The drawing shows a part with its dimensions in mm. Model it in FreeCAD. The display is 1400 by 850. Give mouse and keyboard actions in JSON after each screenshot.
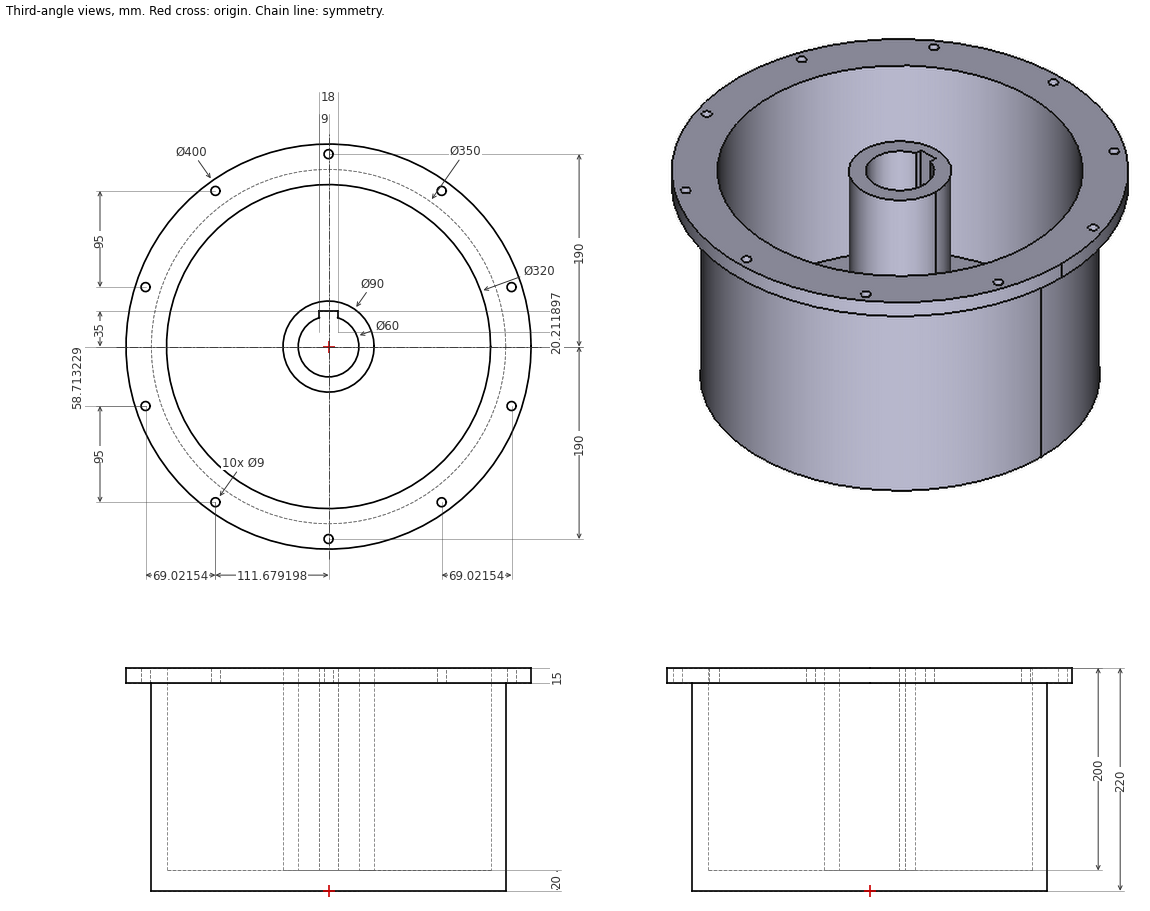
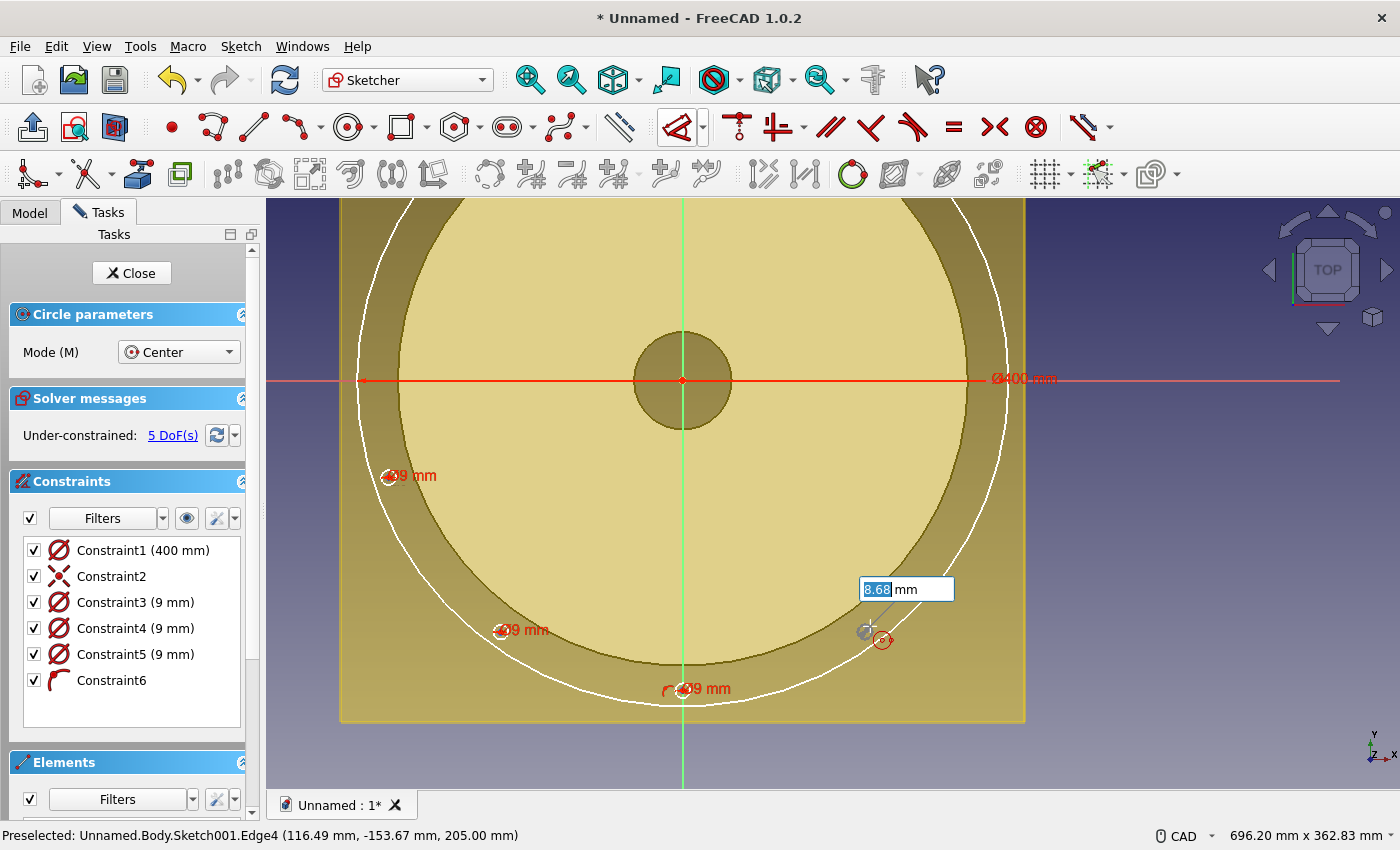
{"action": "type", "text": "9"}
{"action": "key", "text": "Return"}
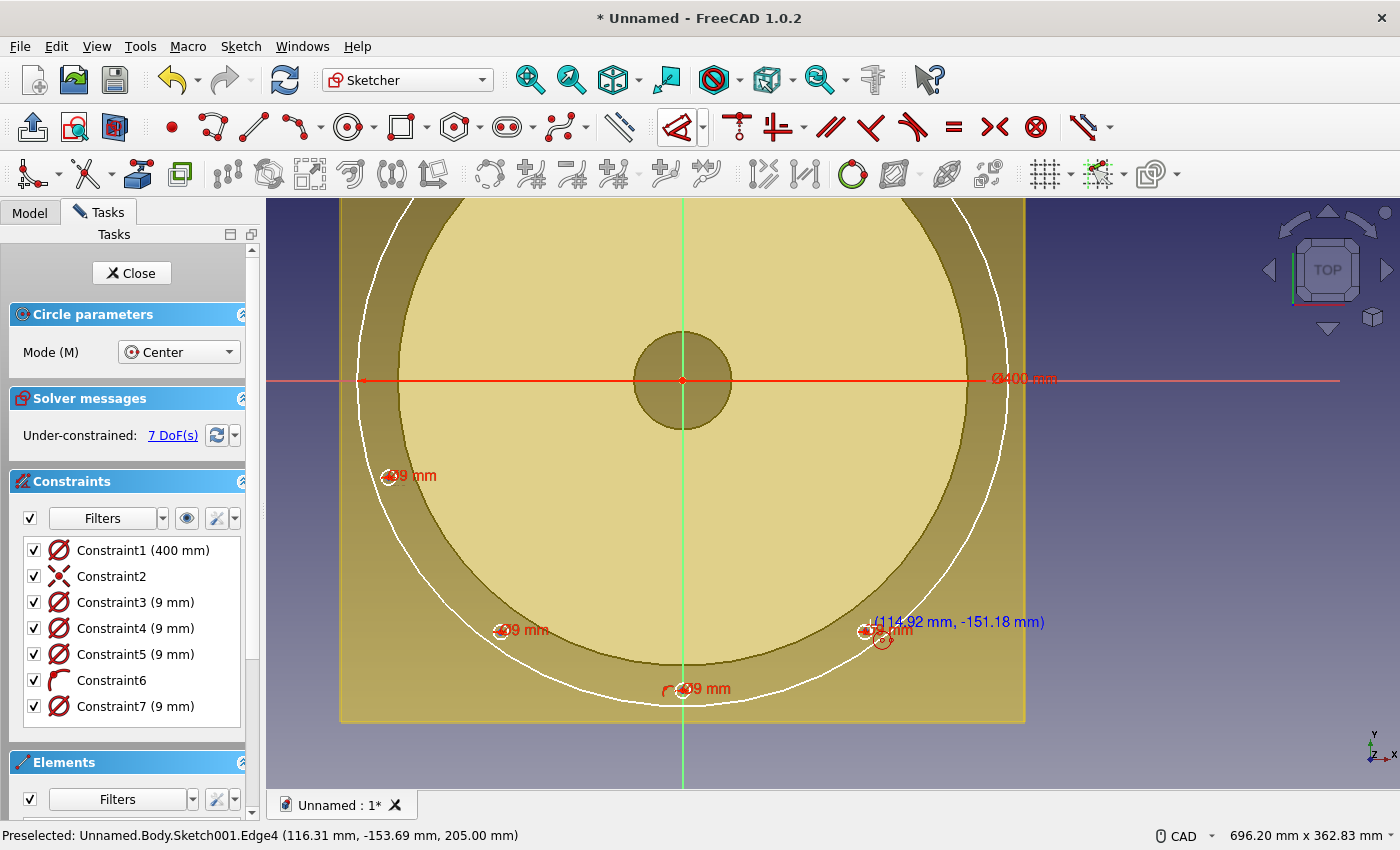
{"action": "left_click", "coordinate": [683, 381]}
{"action": "mouse_move", "coordinate": [717, 346]}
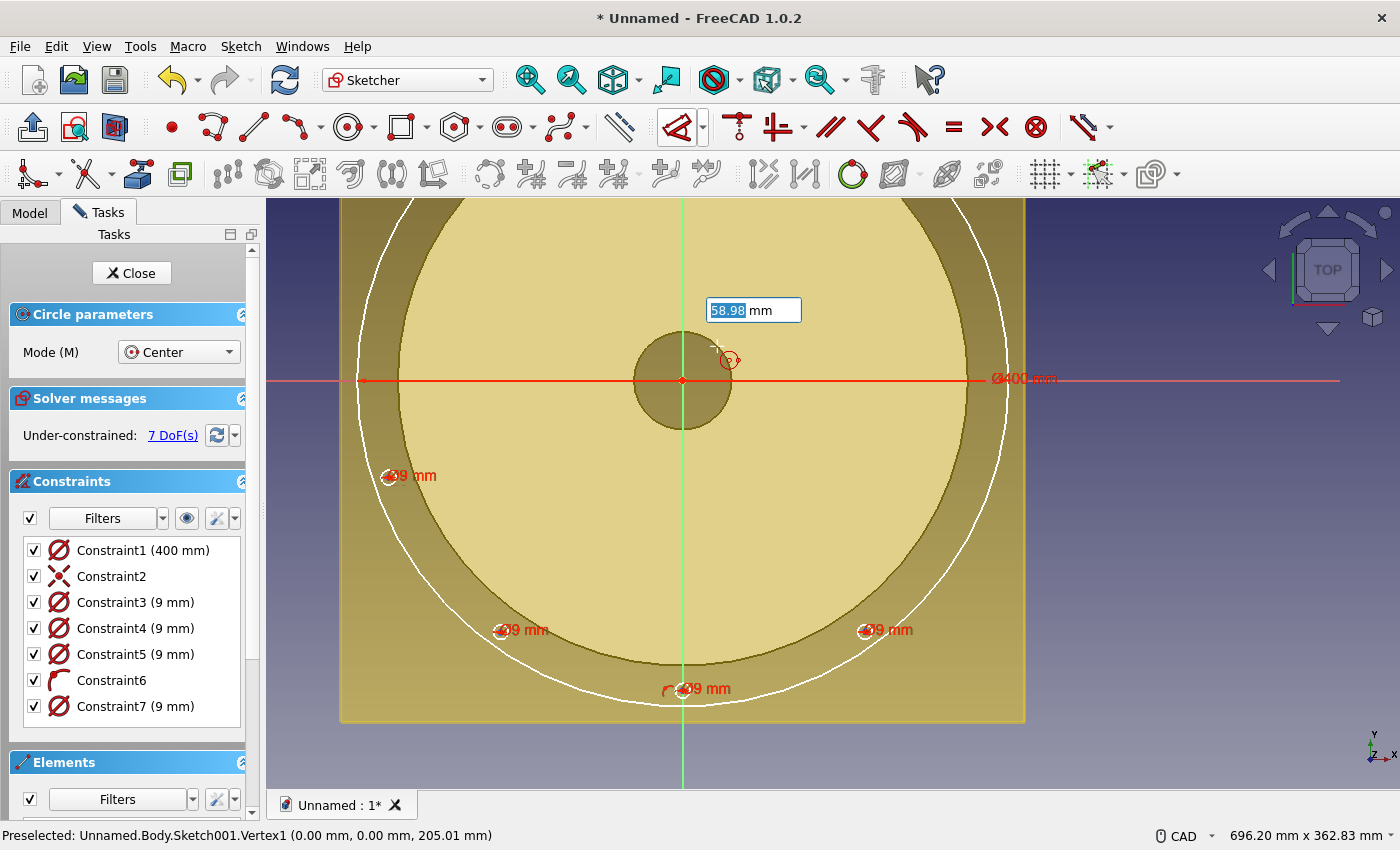
{"action": "type", "text": "60"}
{"action": "key", "text": "Return"}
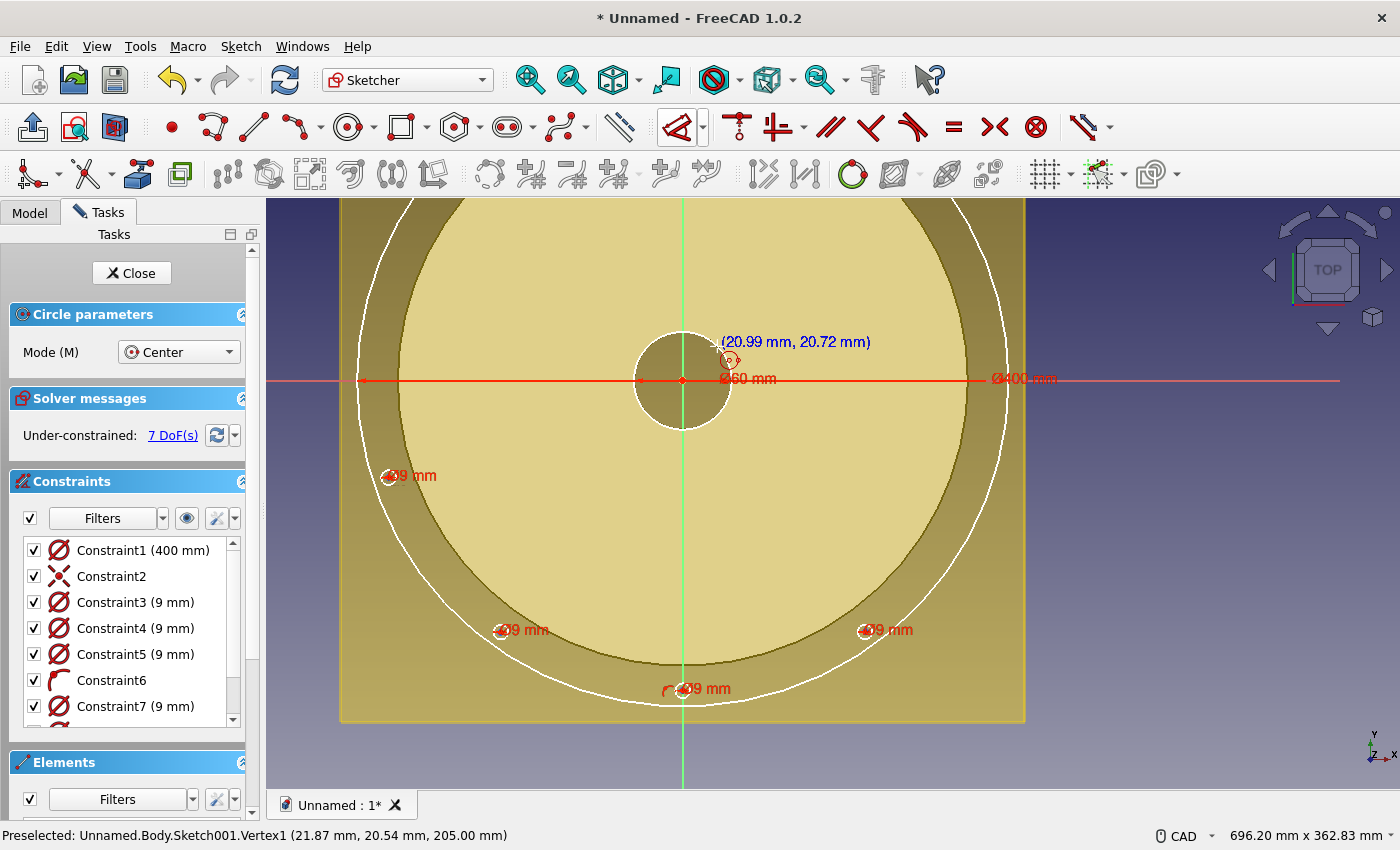
{"action": "scroll", "coordinate": [977, 476], "scroll_direction": "up", "scroll_amount": 6}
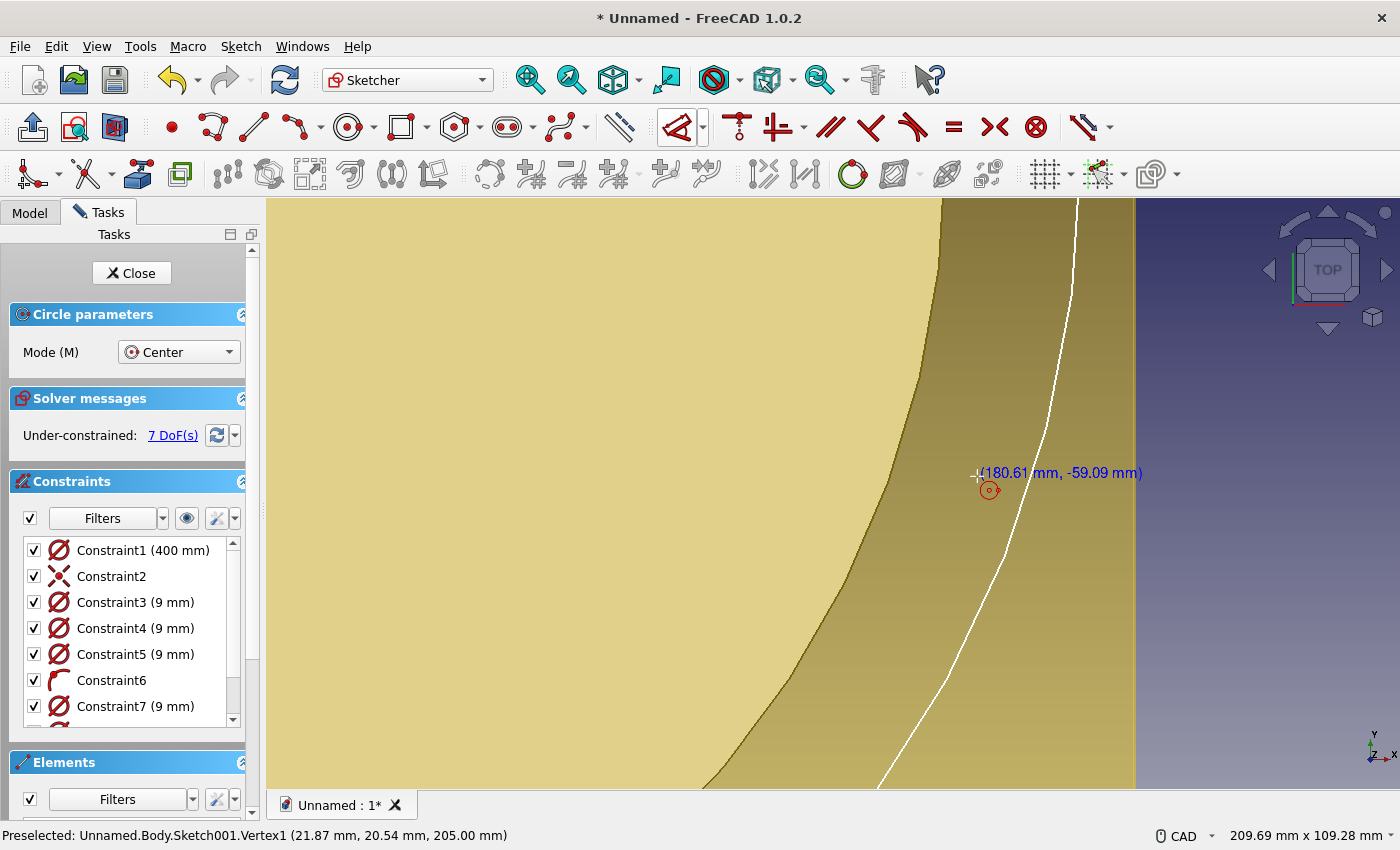
{"action": "scroll", "coordinate": [916, 560], "scroll_direction": "down", "scroll_amount": 9}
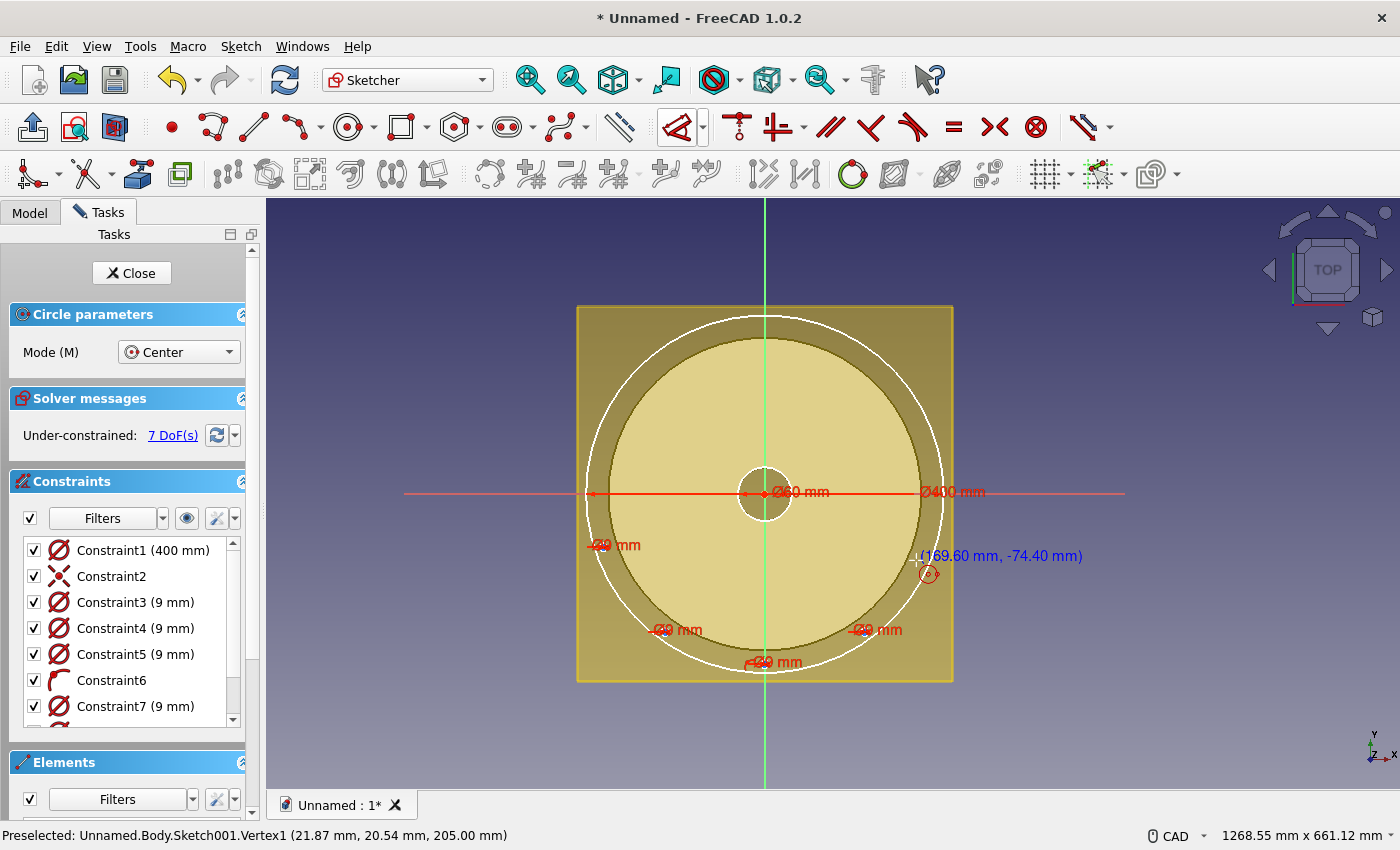
{"action": "scroll", "coordinate": [926, 547], "scroll_direction": "up", "scroll_amount": 3}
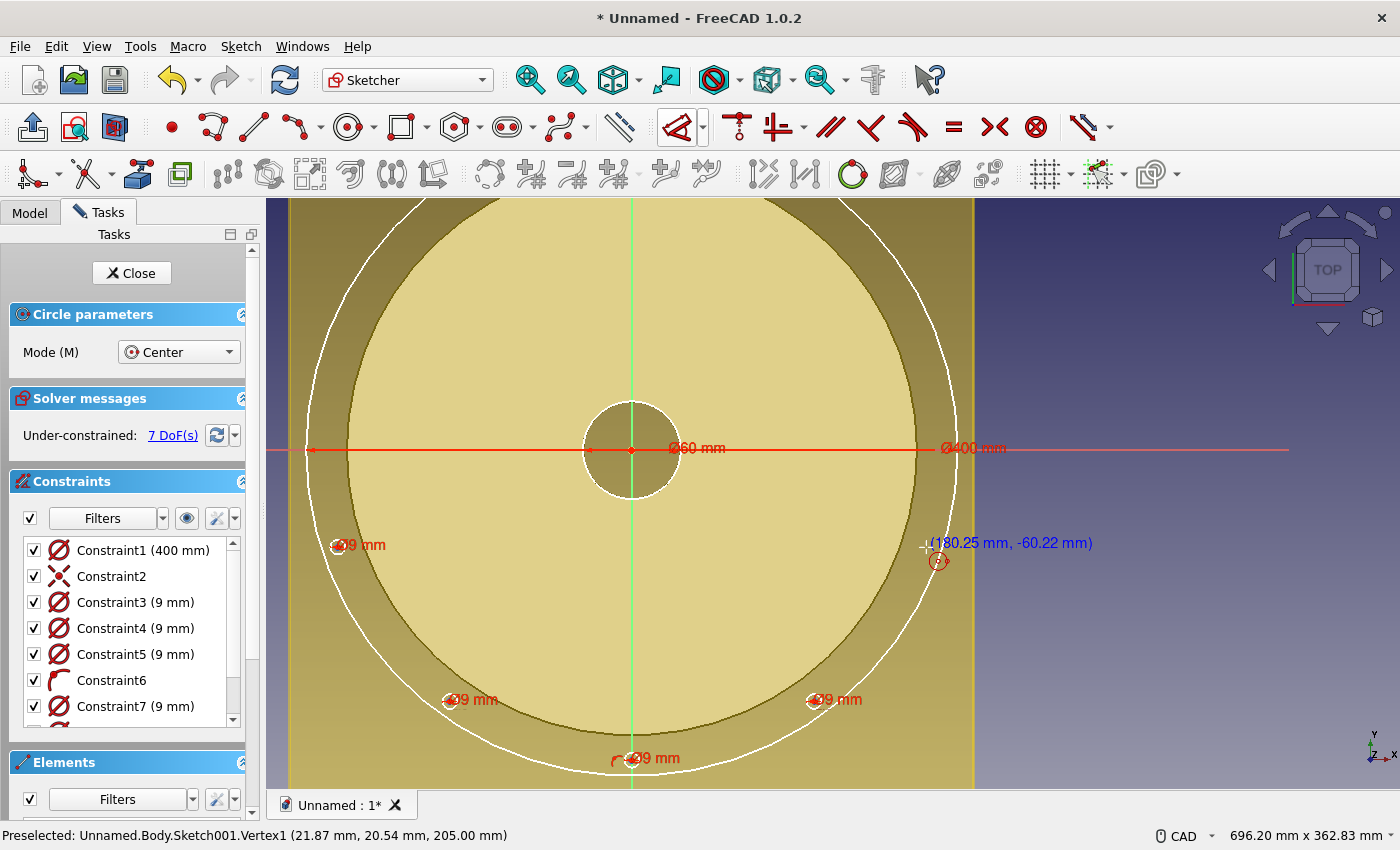
{"action": "left_click", "coordinate": [926, 546]}
{"action": "mouse_move", "coordinate": [921, 541]}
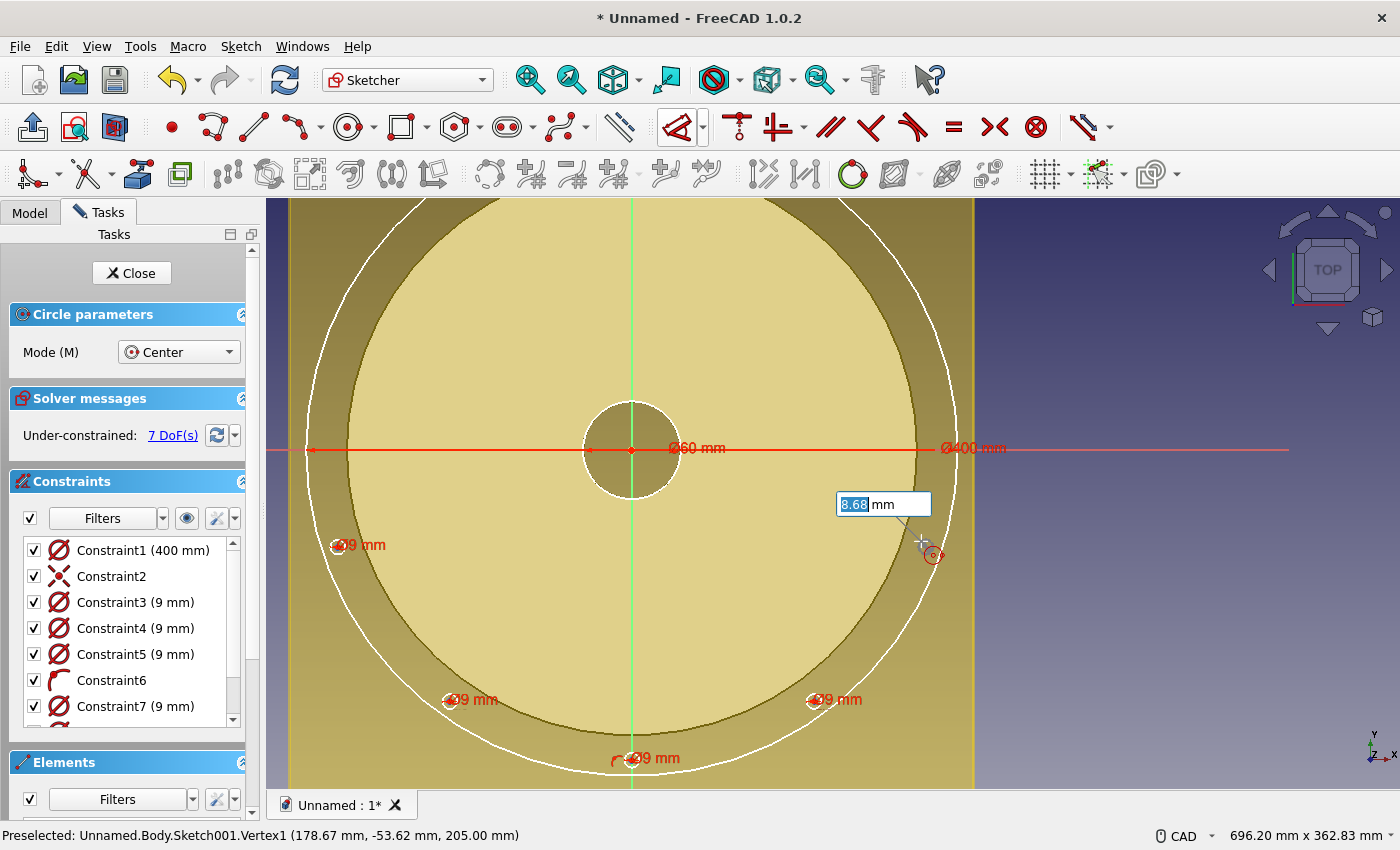
{"action": "type", "text": "9"}
{"action": "key", "text": "Return"}